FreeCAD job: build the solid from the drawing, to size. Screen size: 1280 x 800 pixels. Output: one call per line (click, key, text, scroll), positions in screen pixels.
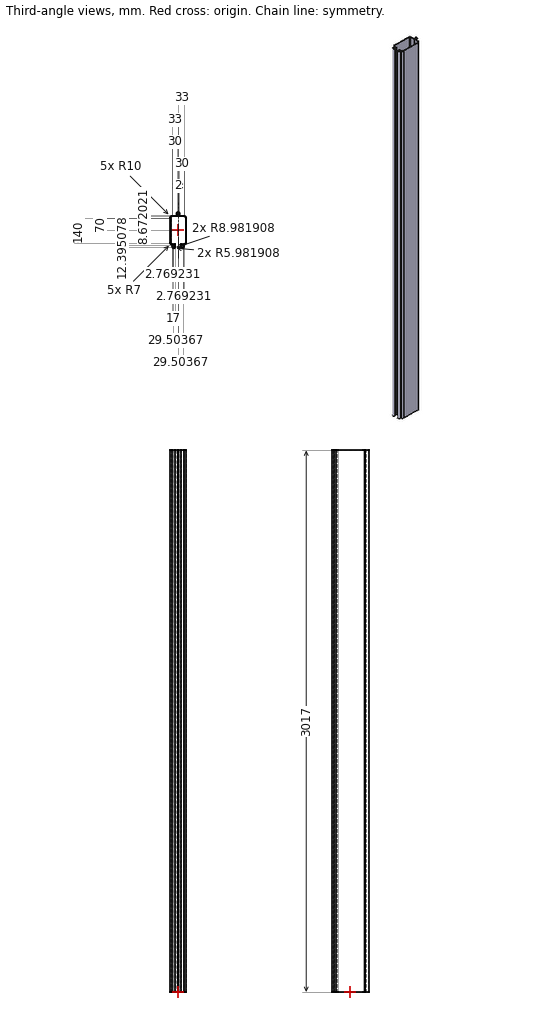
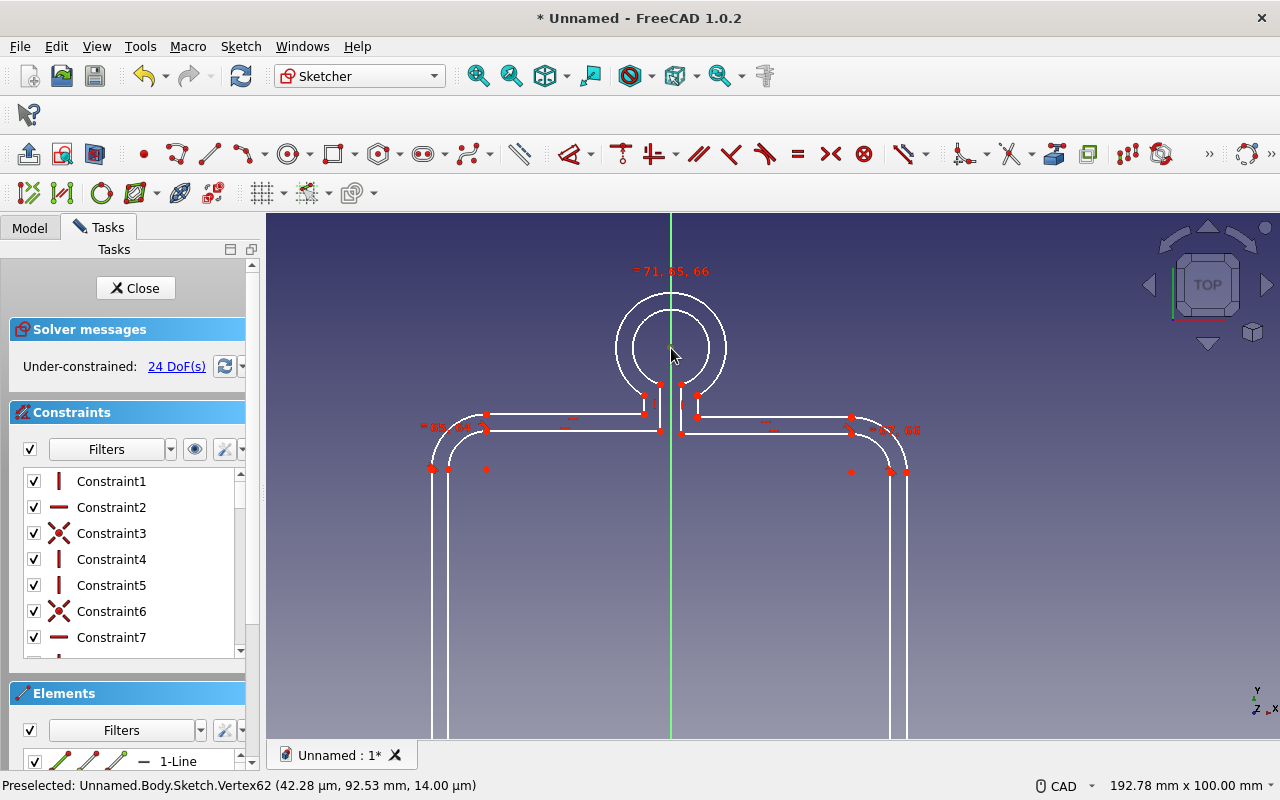
click(671, 677)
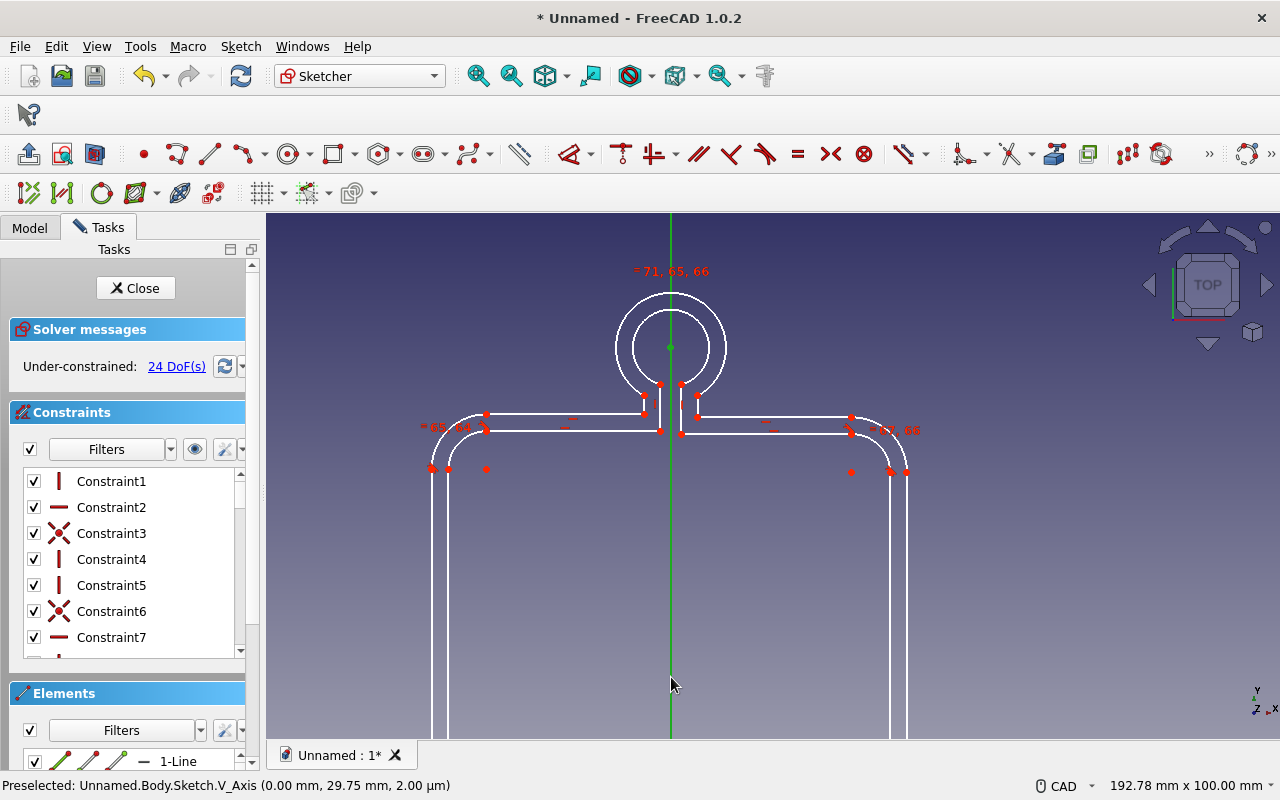
click(621, 154)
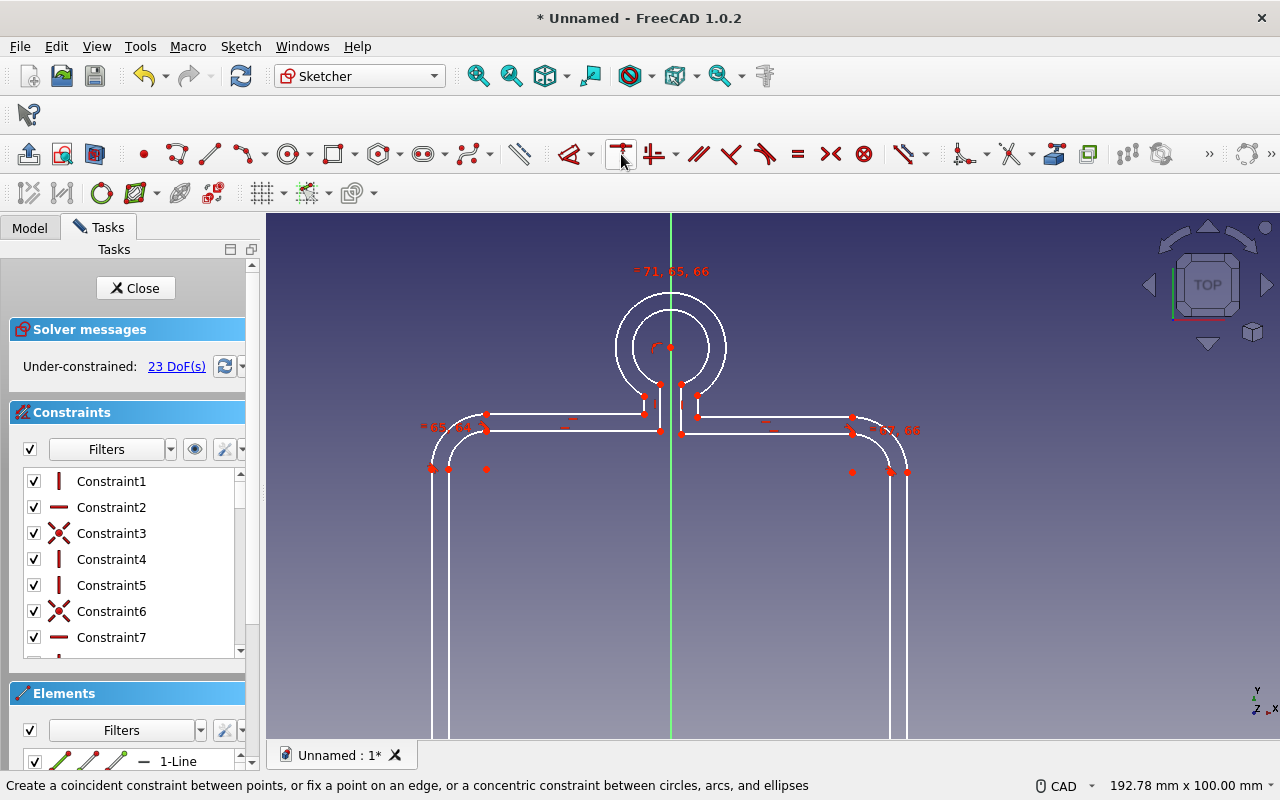
click(487, 469)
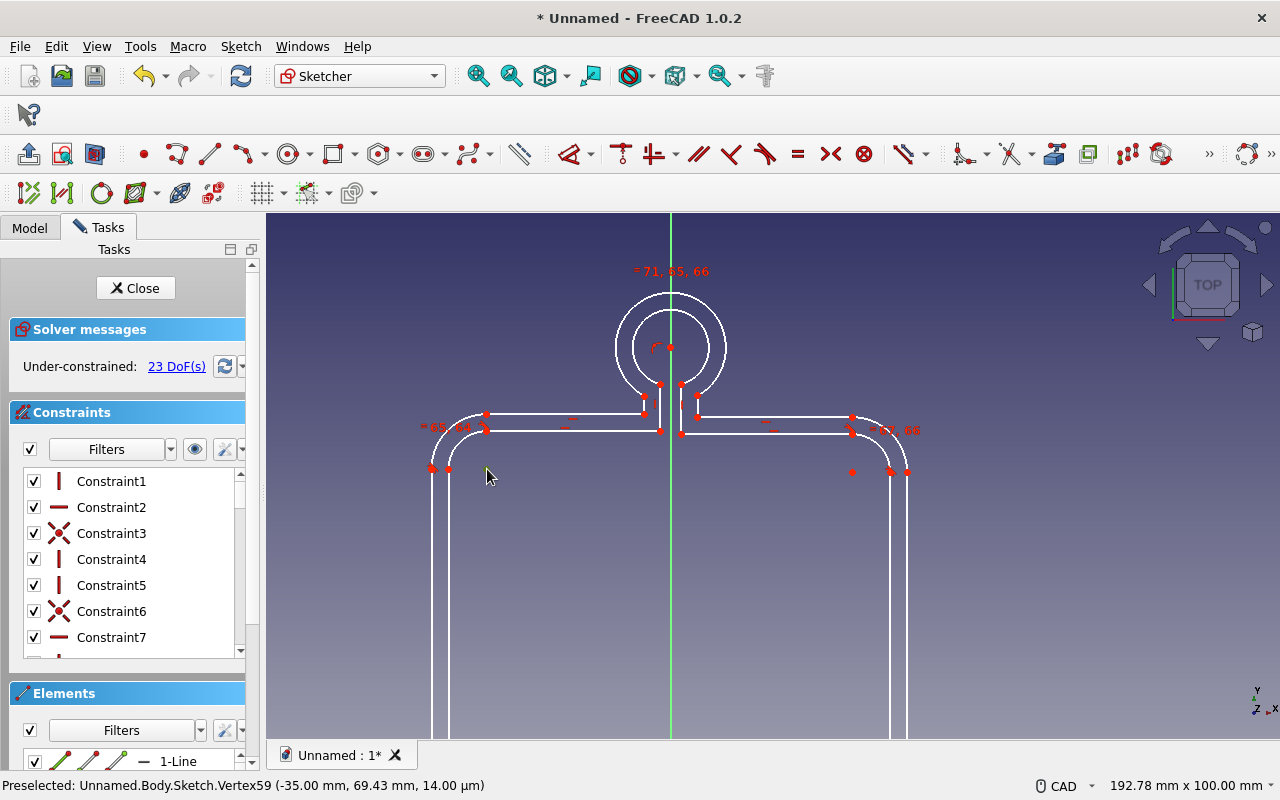
click(852, 472)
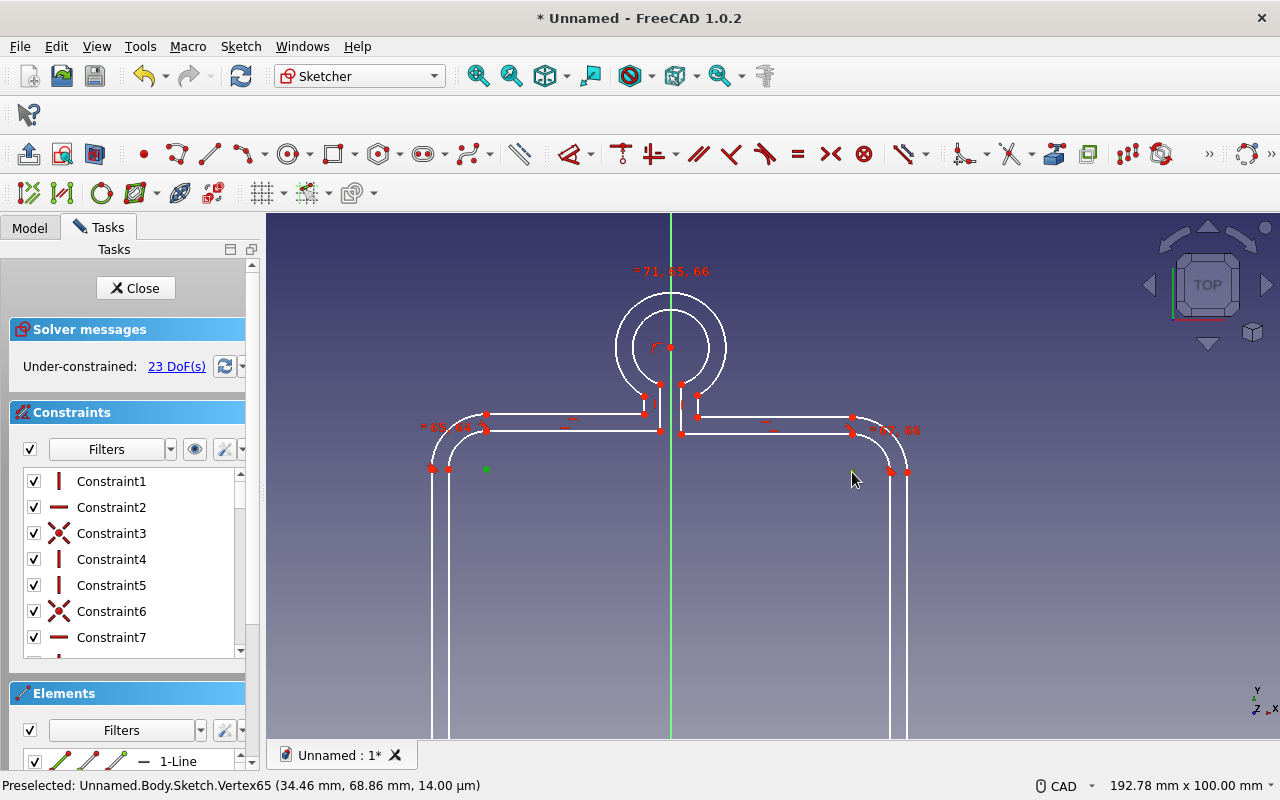
click(671, 677)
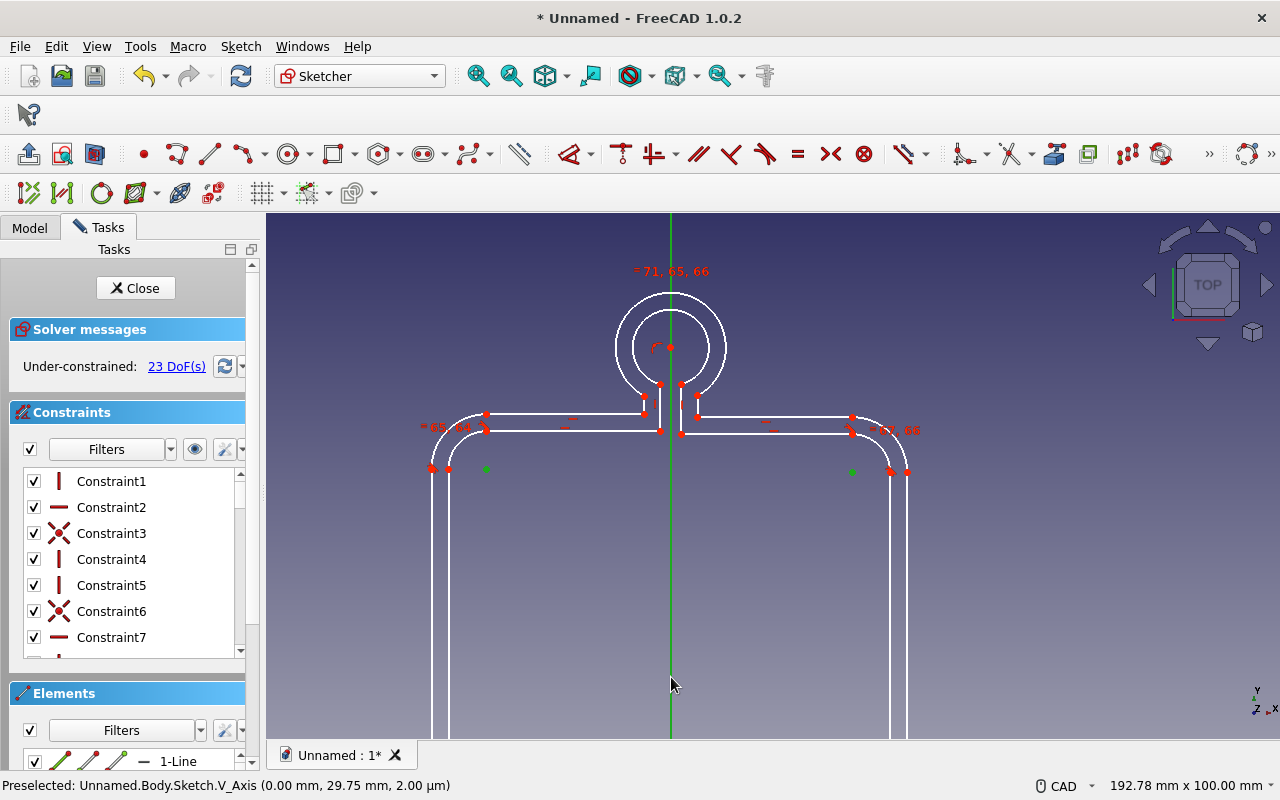
click(831, 154)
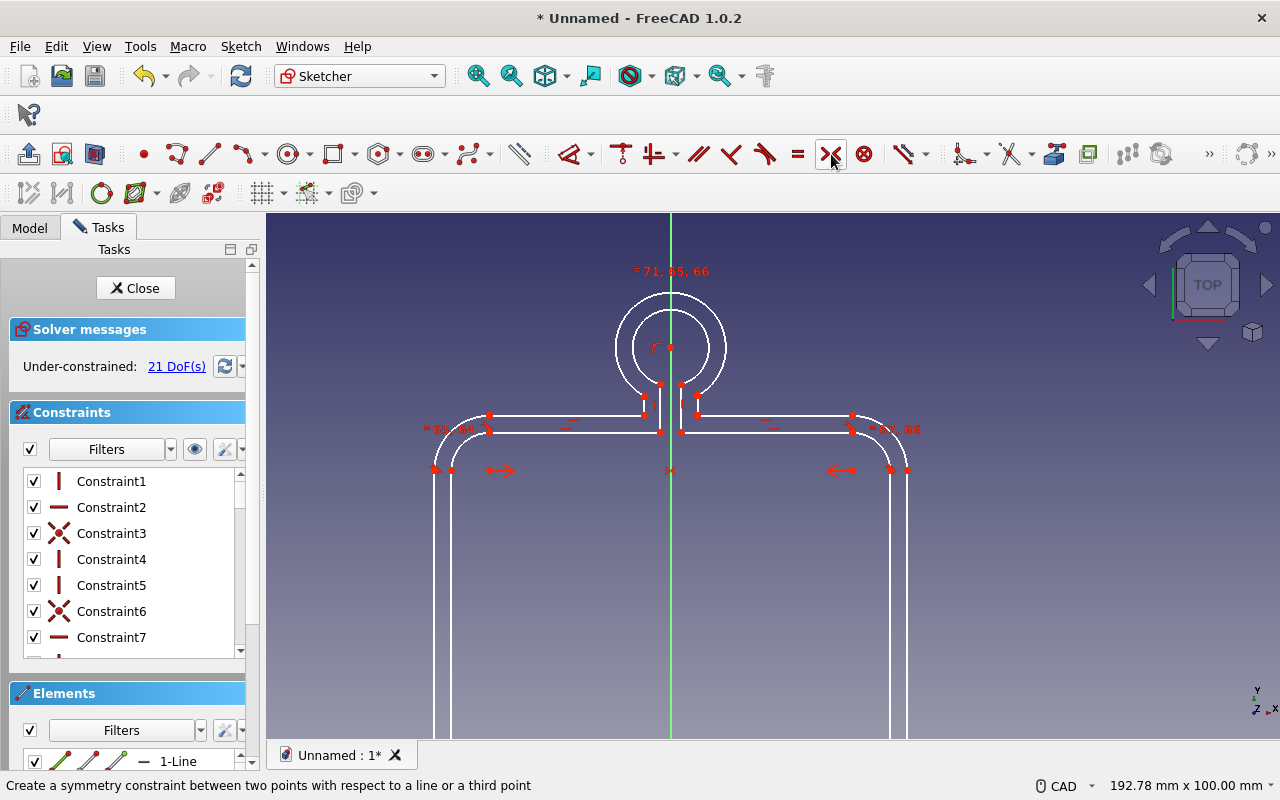
scroll(719, 323, down, 6)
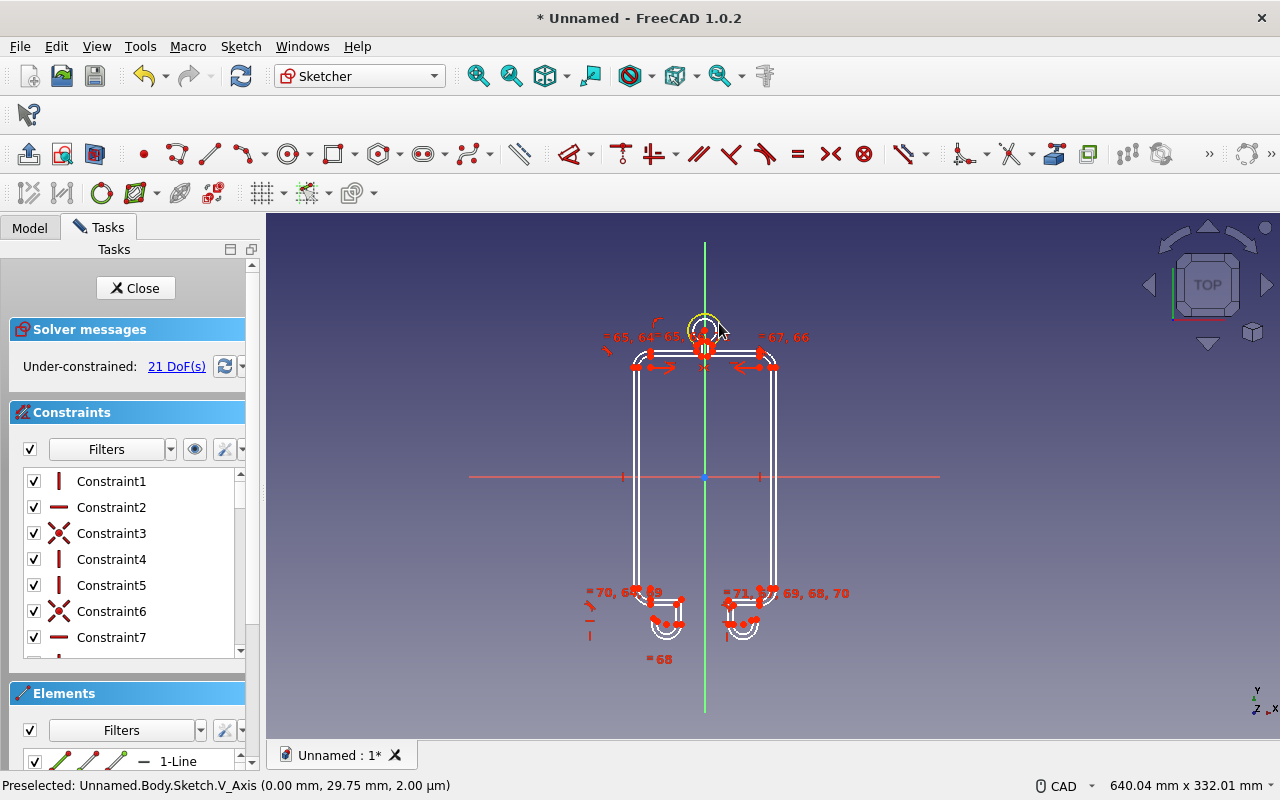
scroll(667, 625, up, 2)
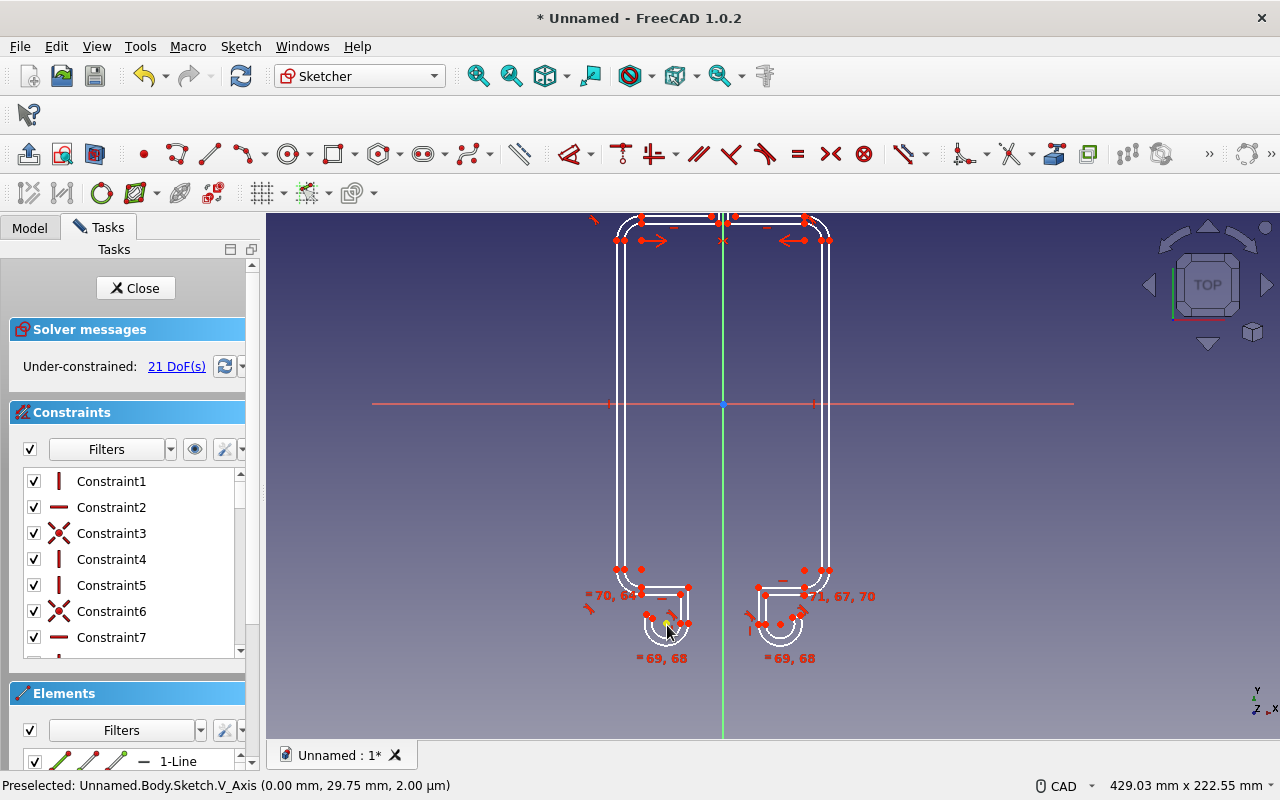
click(666, 624)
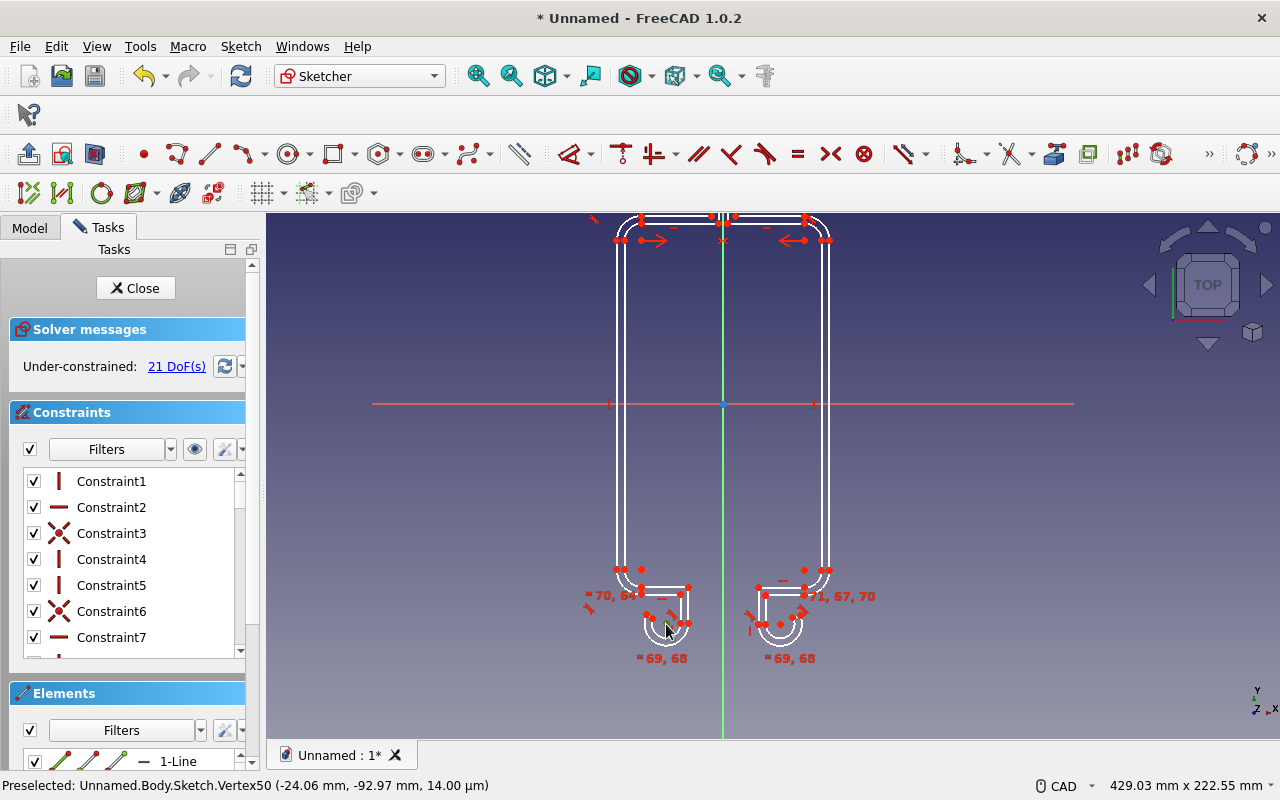
click(780, 624)